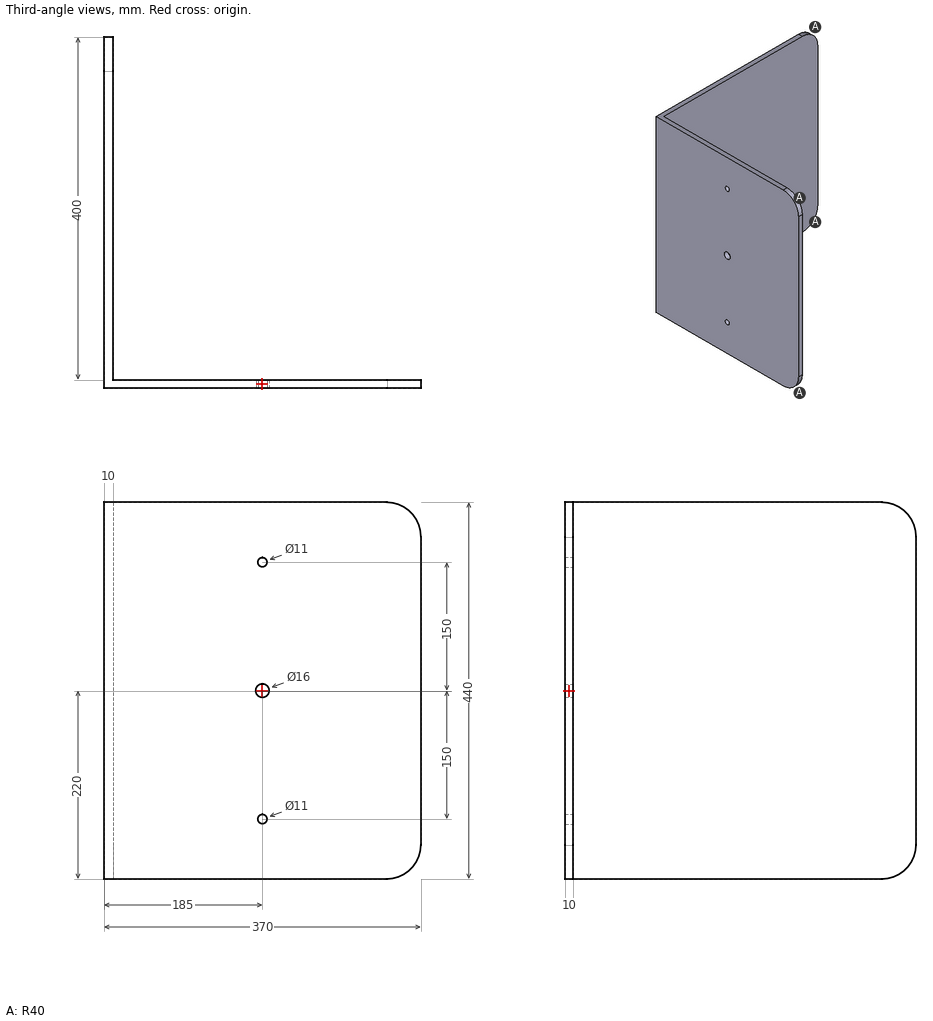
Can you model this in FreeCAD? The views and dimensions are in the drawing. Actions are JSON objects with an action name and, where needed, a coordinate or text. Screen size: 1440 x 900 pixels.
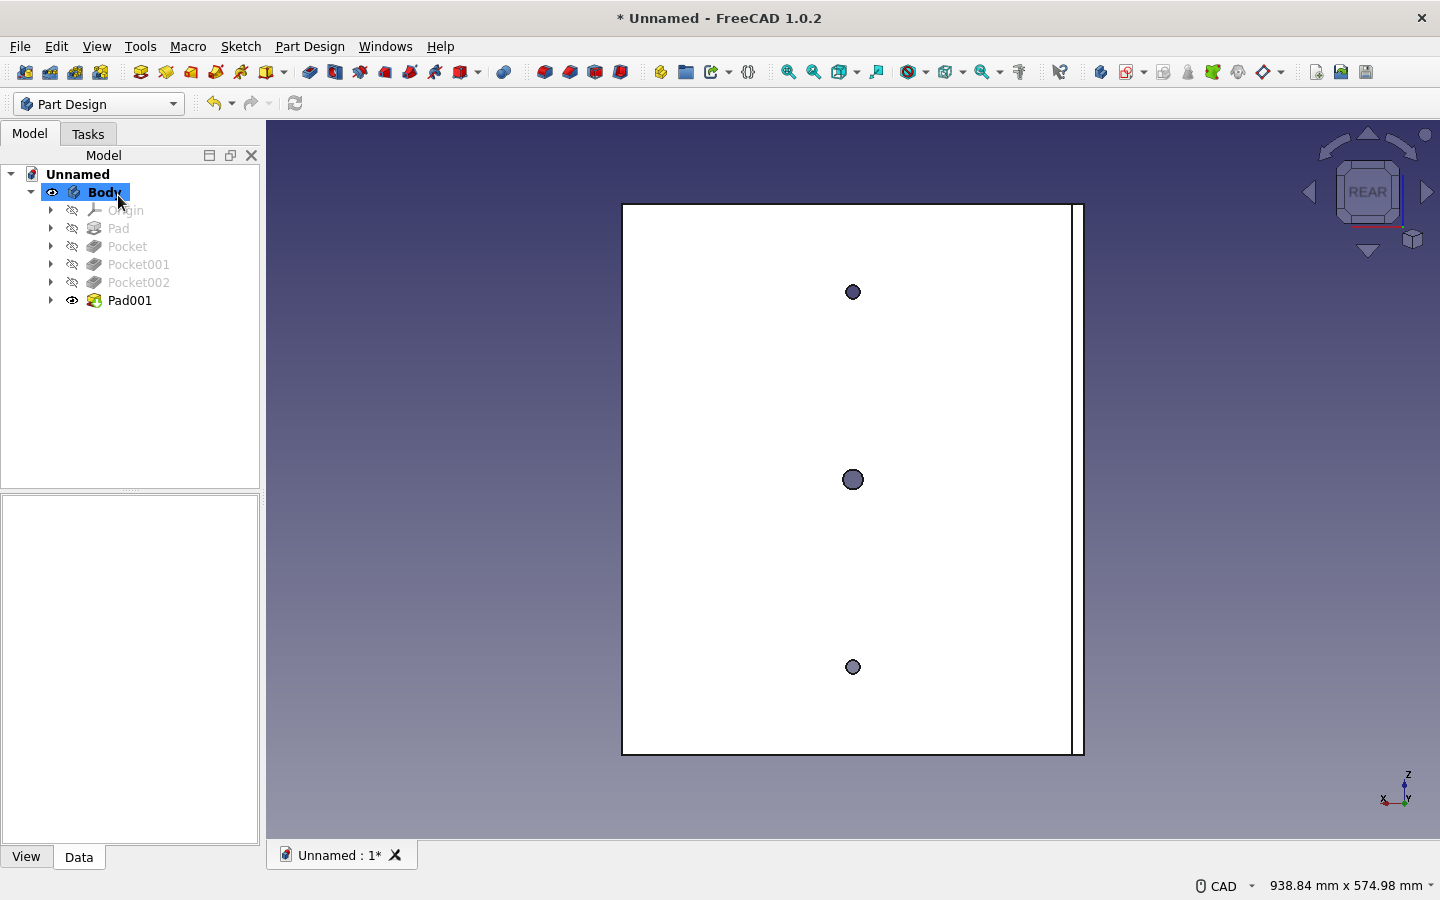
{"action": "left_click", "coordinate": [1078, 754]}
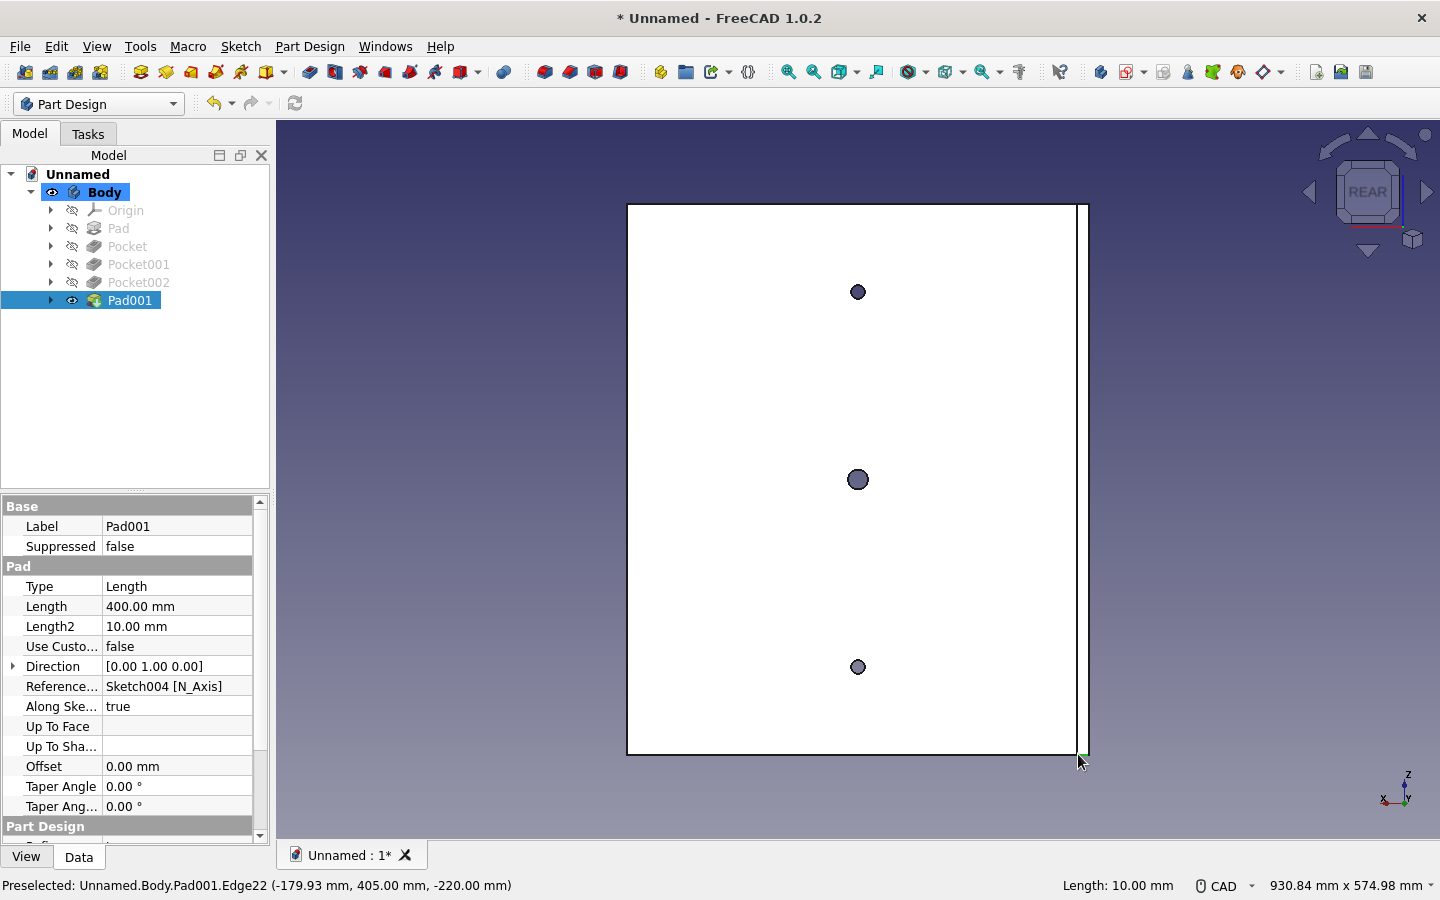
{"action": "scroll", "coordinate": [1083, 203], "scroll_direction": "up", "scroll_amount": 6}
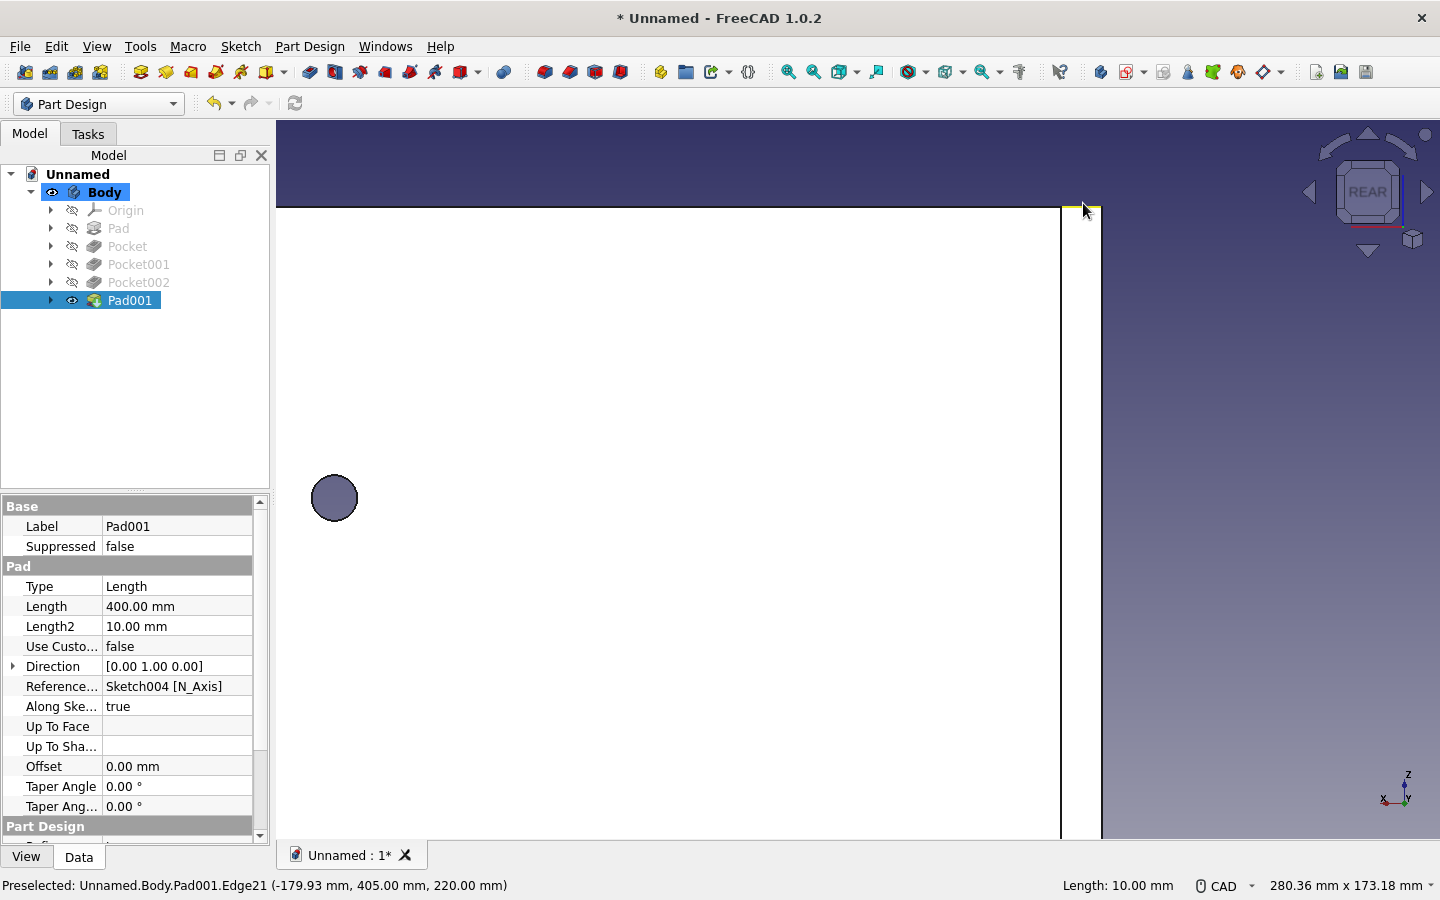
{"action": "left_click", "coordinate": [789, 72]}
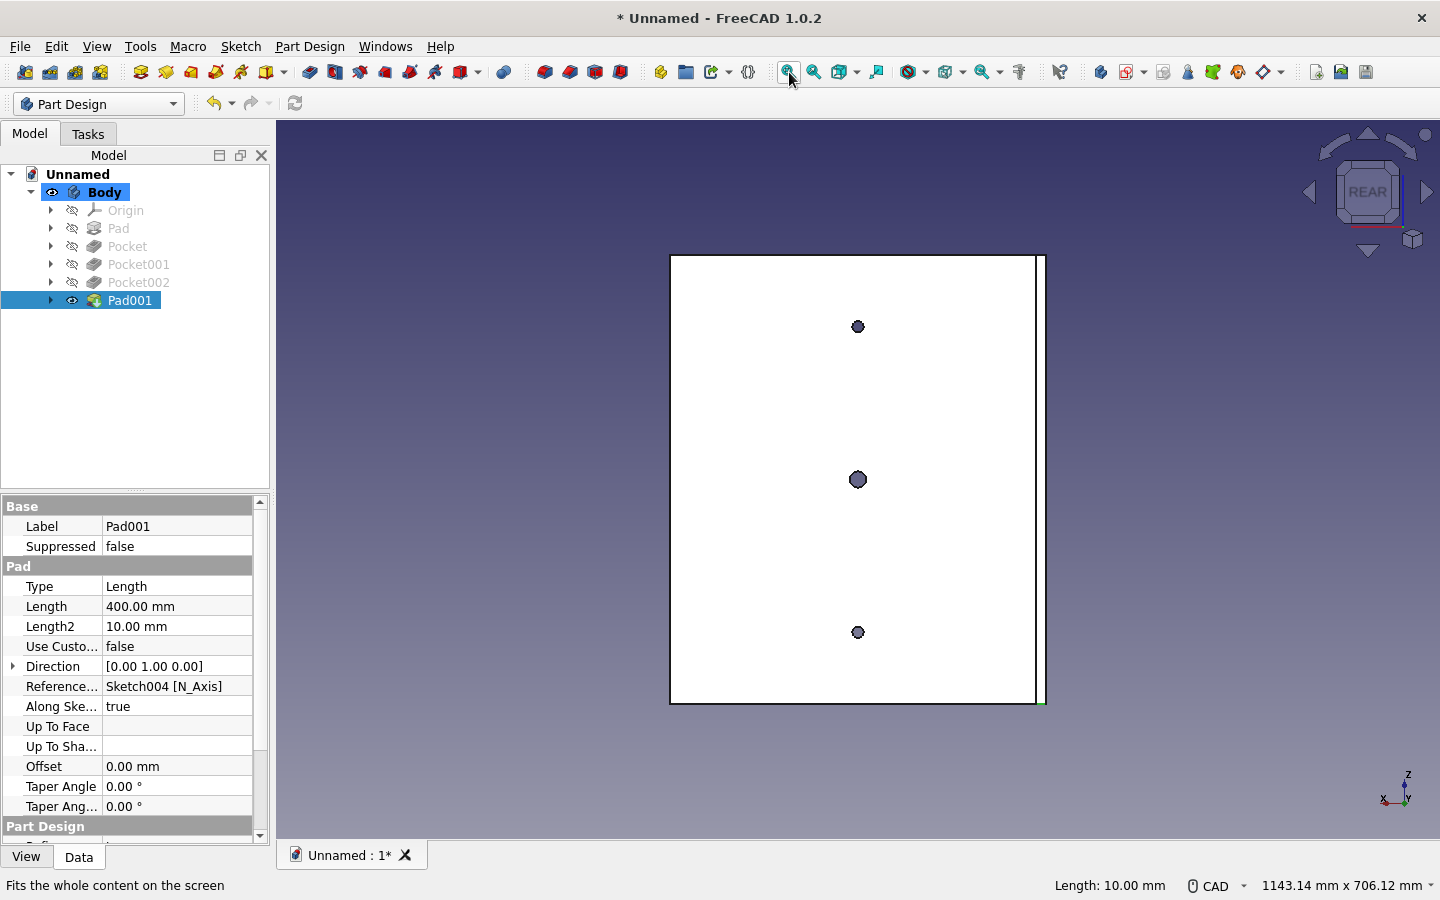
{"action": "key", "text": "0"}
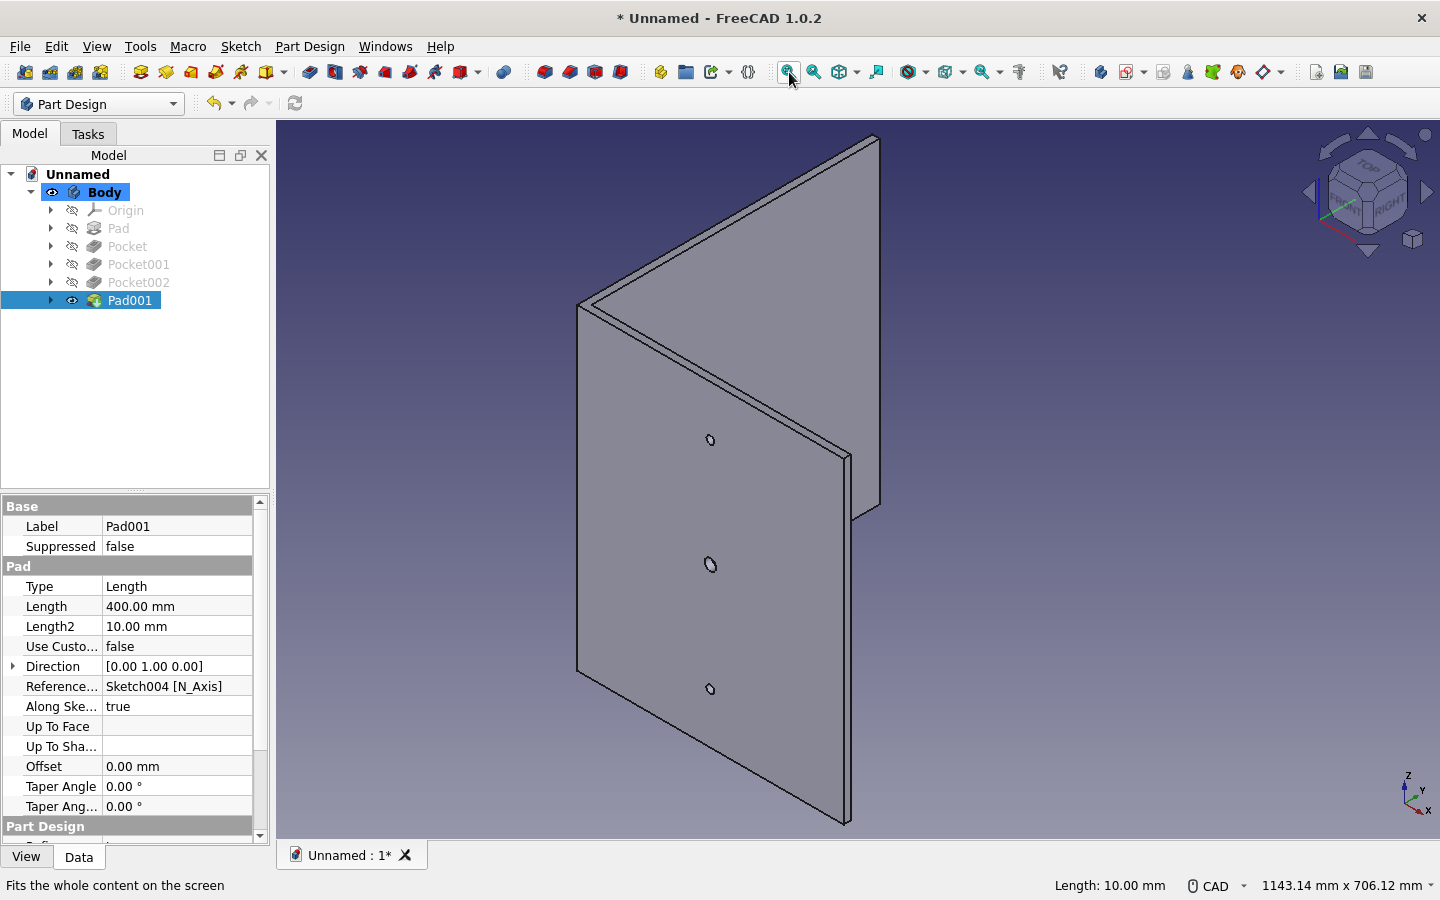
{"action": "left_click", "coordinate": [849, 454], "text": "ctrl"}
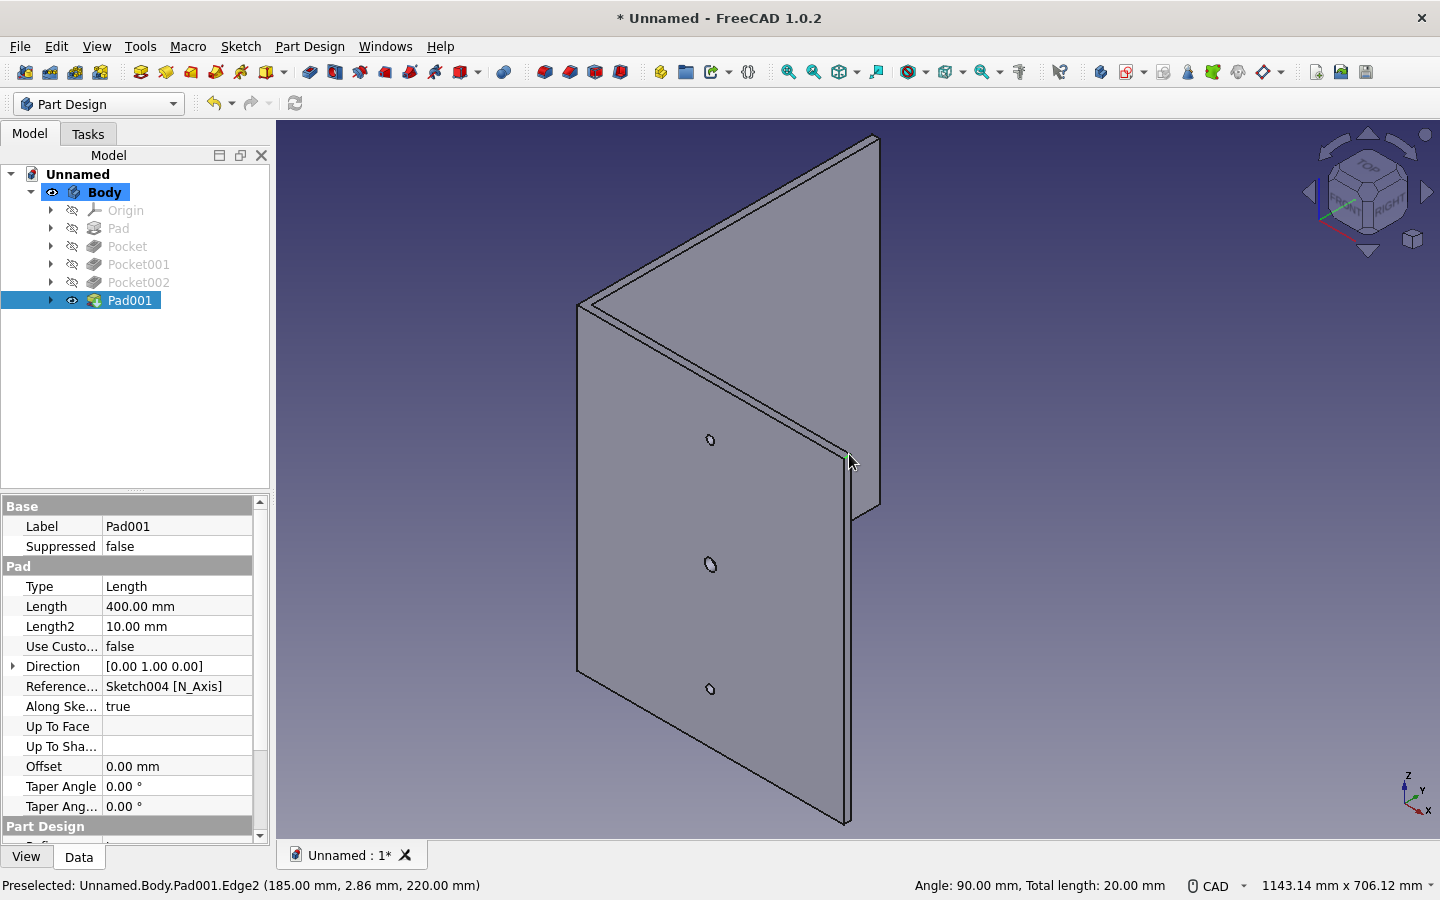
{"action": "key", "text": "2"}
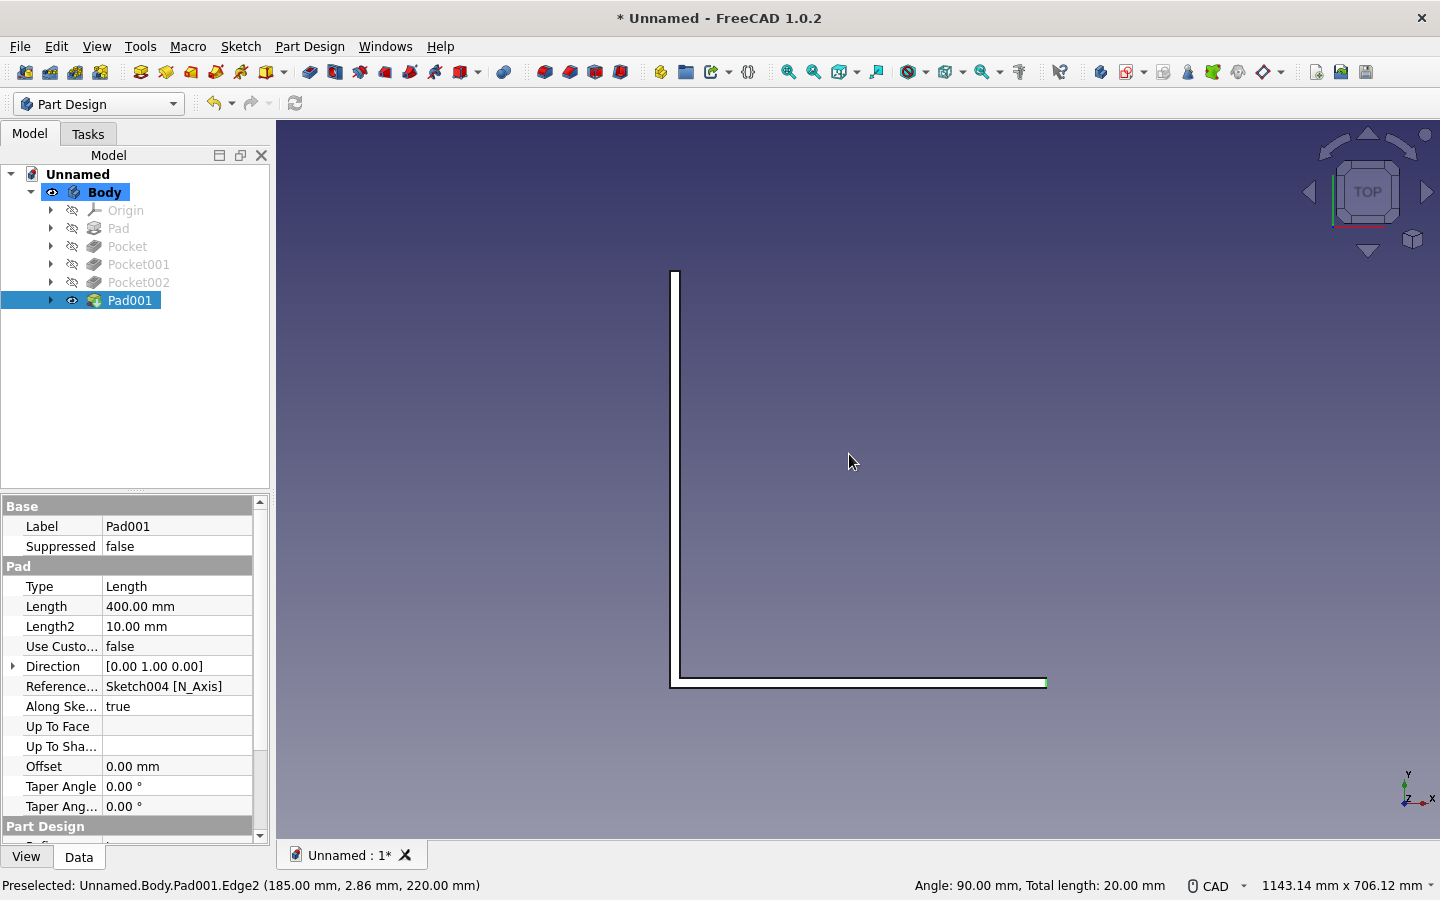
{"action": "scroll", "coordinate": [675, 270], "scroll_direction": "up", "scroll_amount": 7}